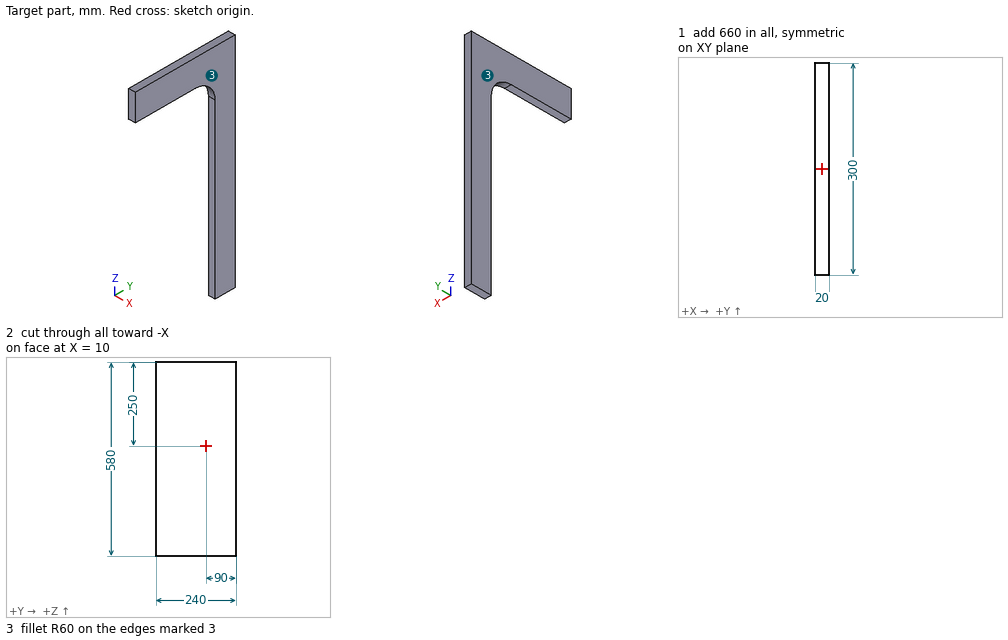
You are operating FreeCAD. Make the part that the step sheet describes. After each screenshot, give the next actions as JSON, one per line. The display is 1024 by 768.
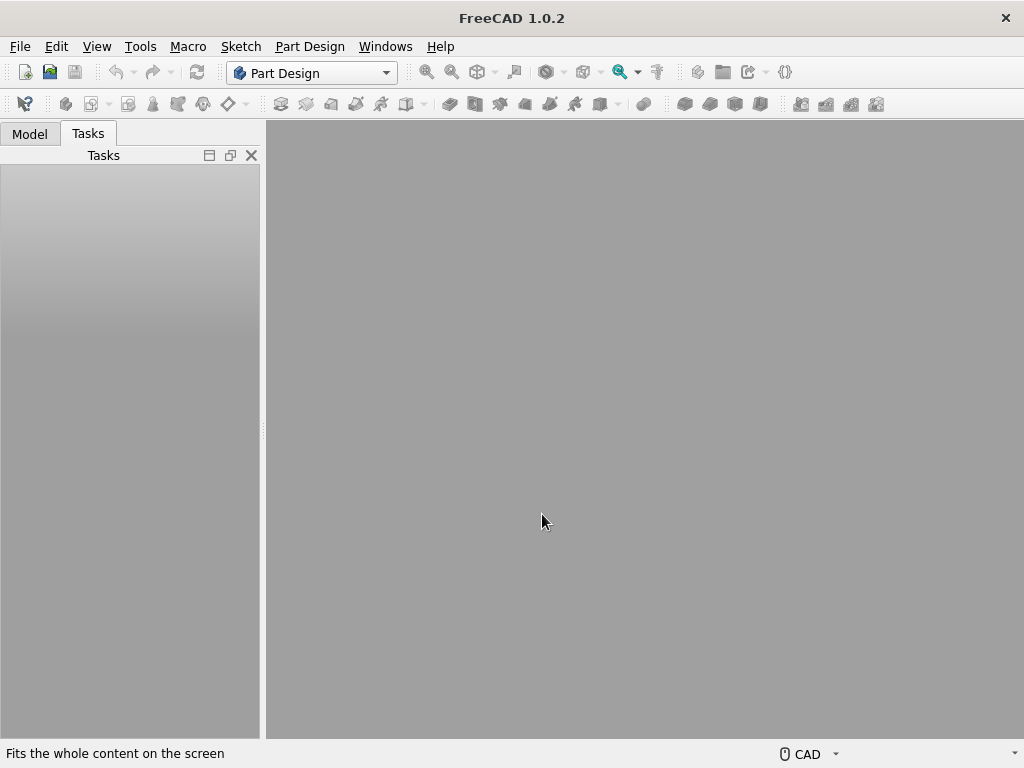
{"action": "key", "text": "ctrl+n"}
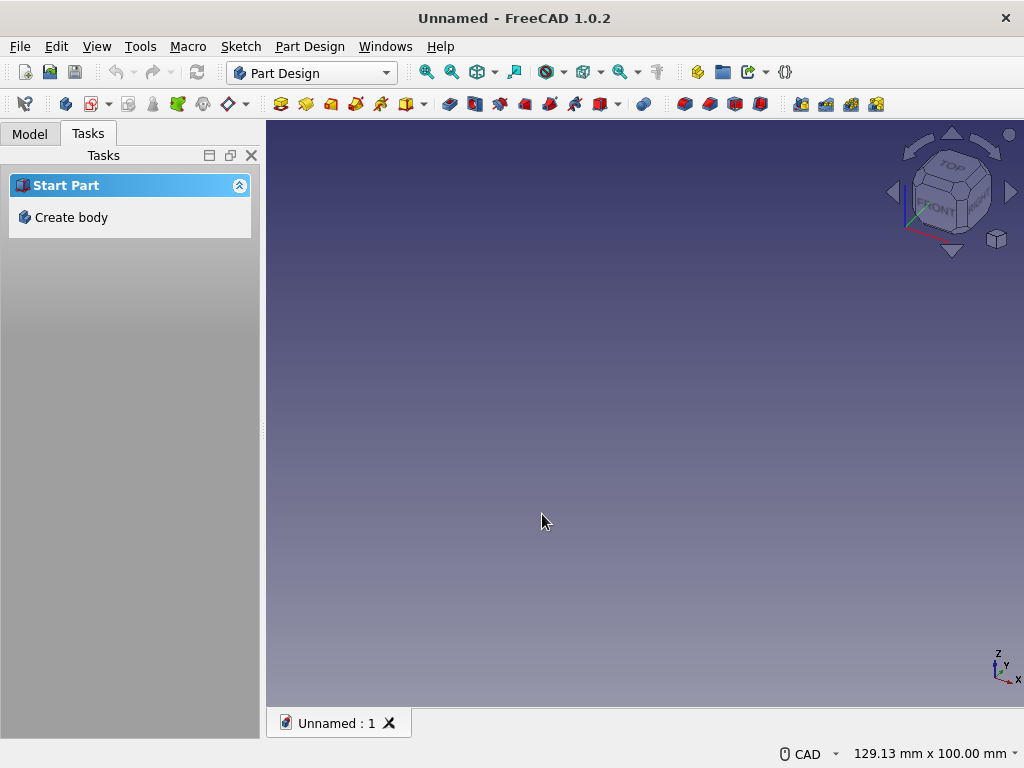
{"action": "left_click", "coordinate": [90, 104]}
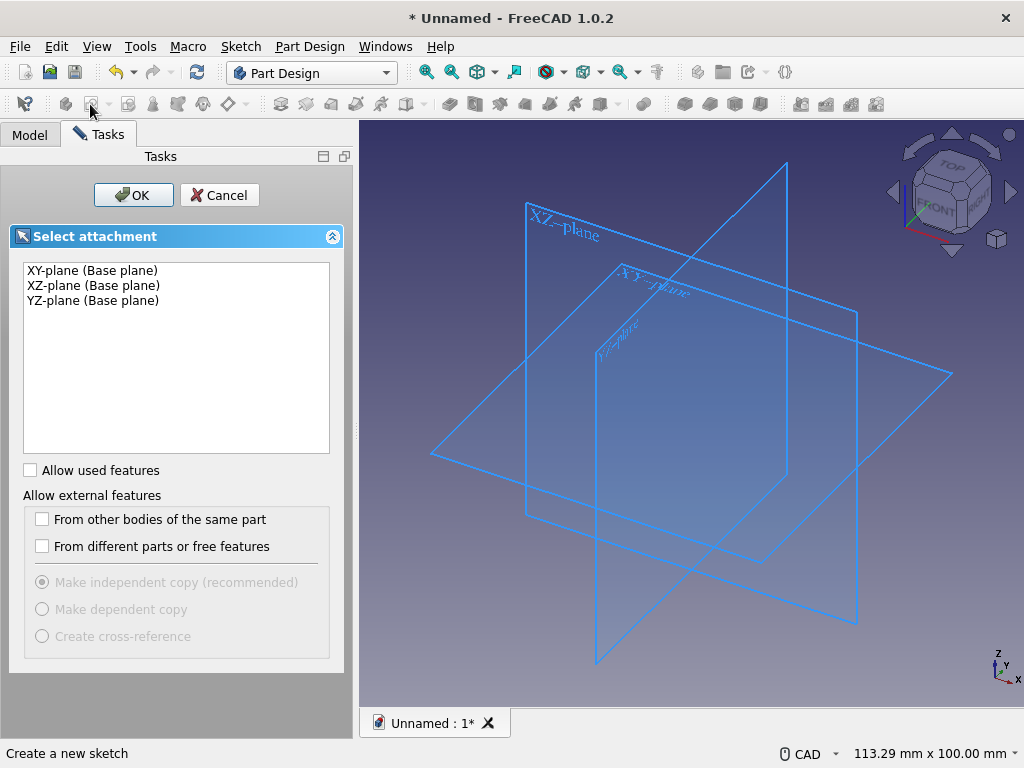
{"action": "left_click", "coordinate": [84, 270]}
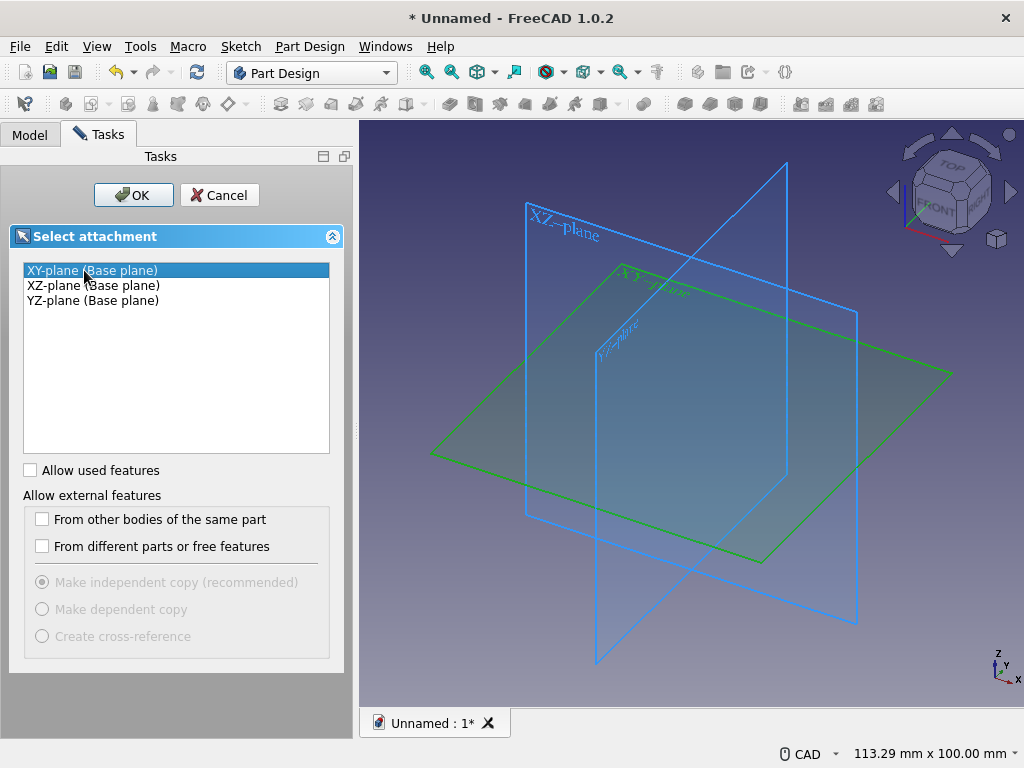
{"action": "left_click", "coordinate": [134, 195]}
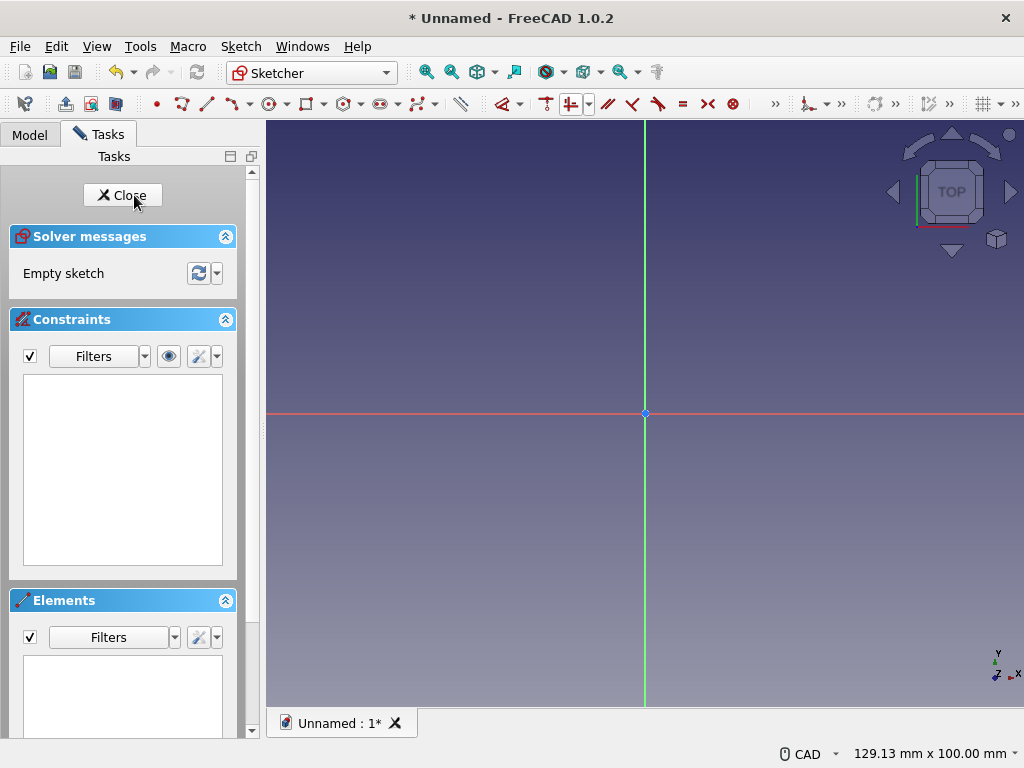
{"action": "scroll", "coordinate": [559, 414], "scroll_direction": "down", "scroll_amount": 8}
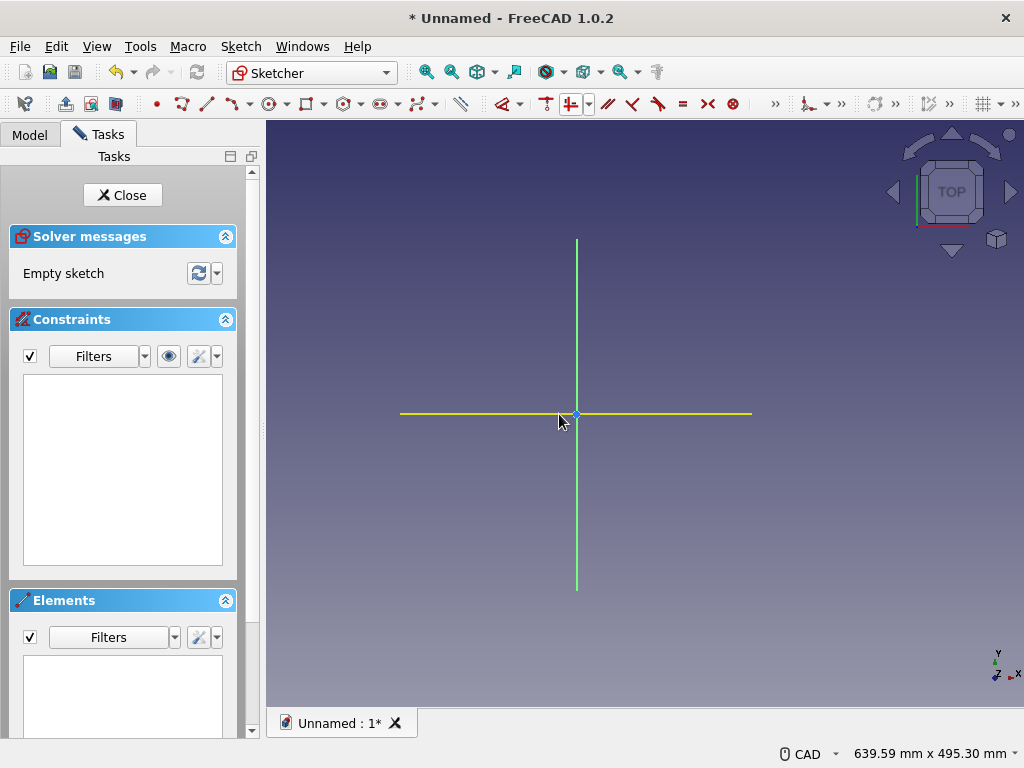
{"action": "left_click", "coordinate": [324, 104]}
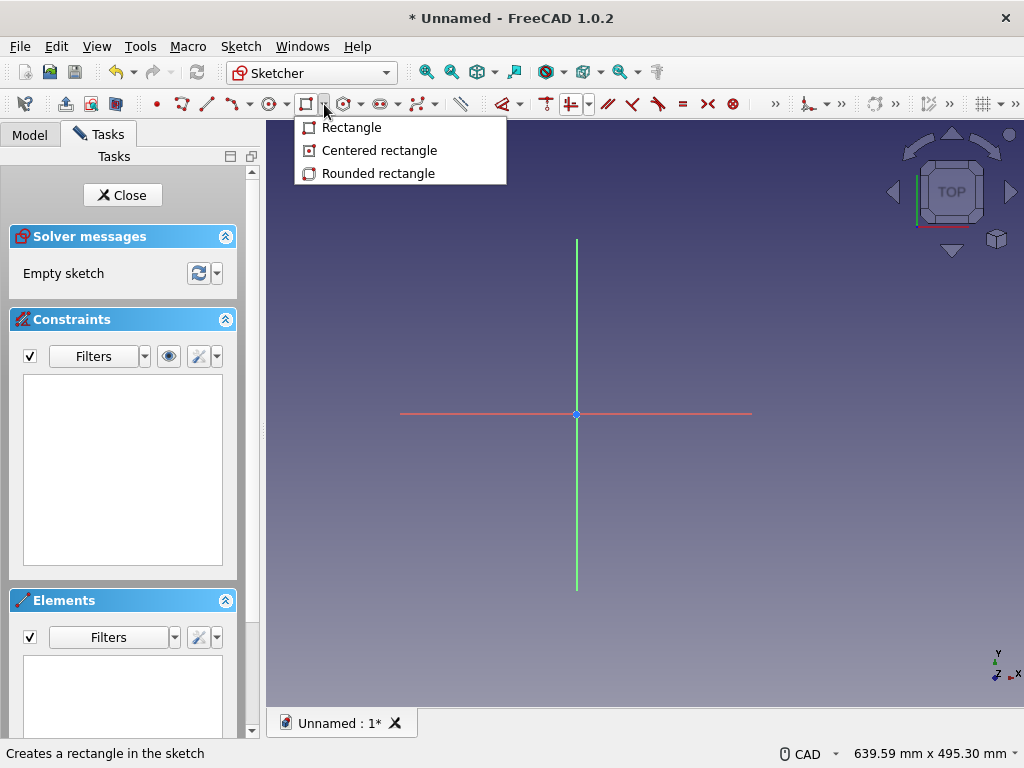
{"action": "left_click", "coordinate": [400, 150]}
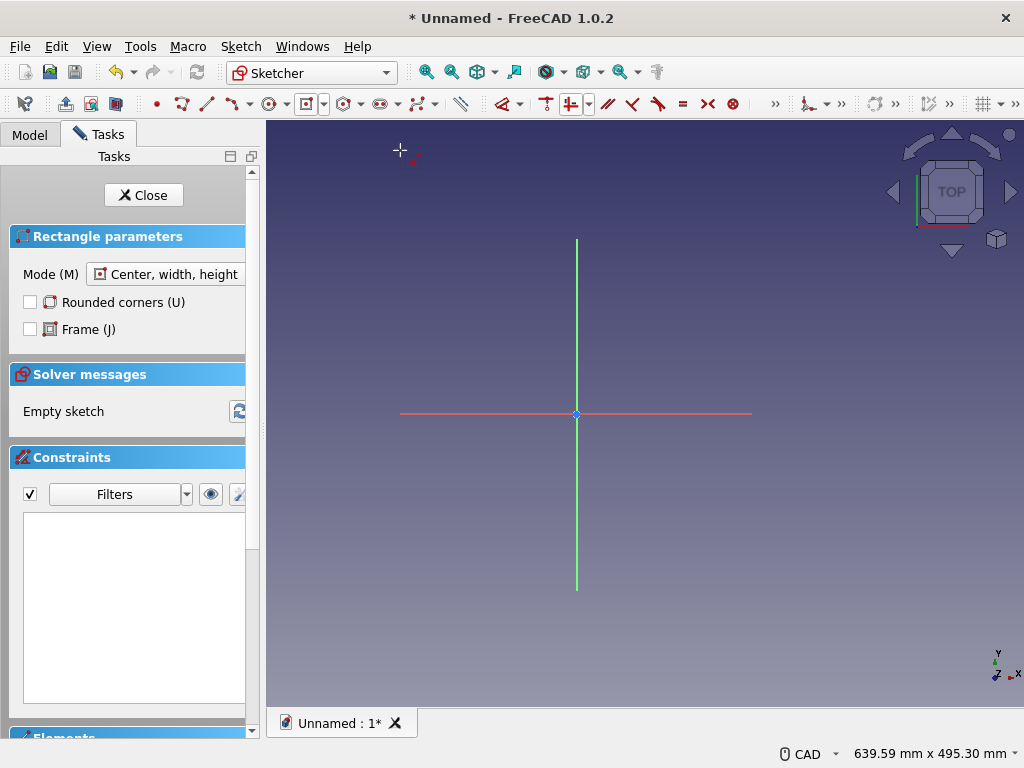
{"action": "scroll", "coordinate": [577, 414], "scroll_direction": "up", "scroll_amount": 2}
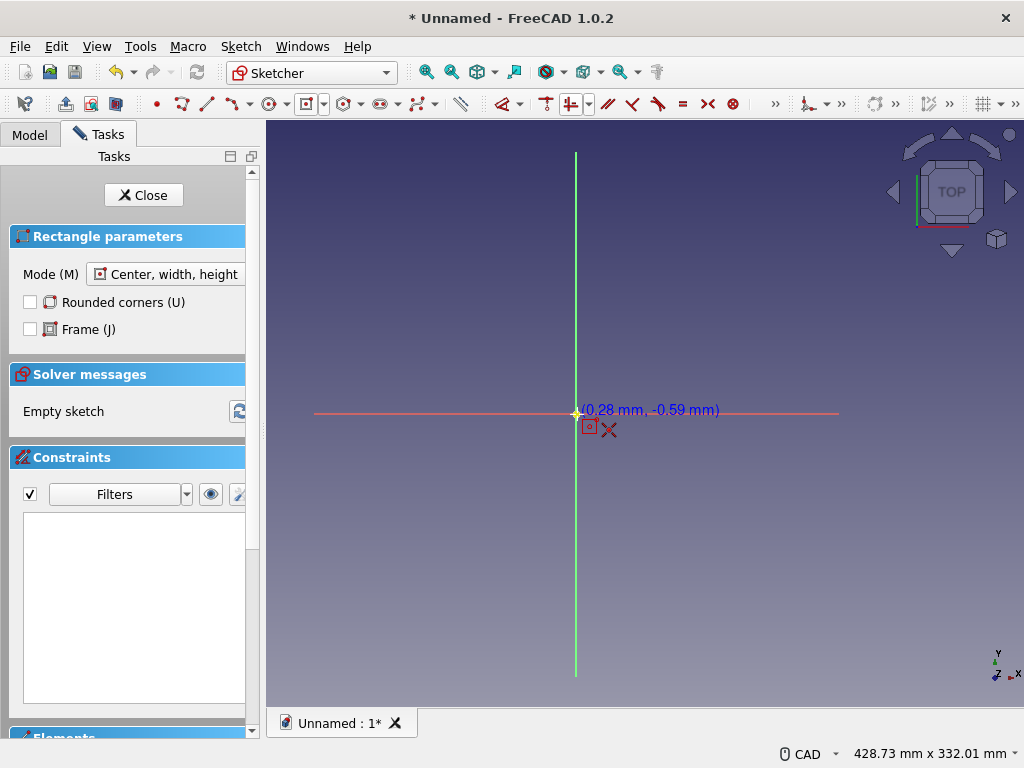
{"action": "left_click", "coordinate": [576, 414]}
{"action": "left_click", "coordinate": [594, 149]}
{"action": "key", "text": "Escape"}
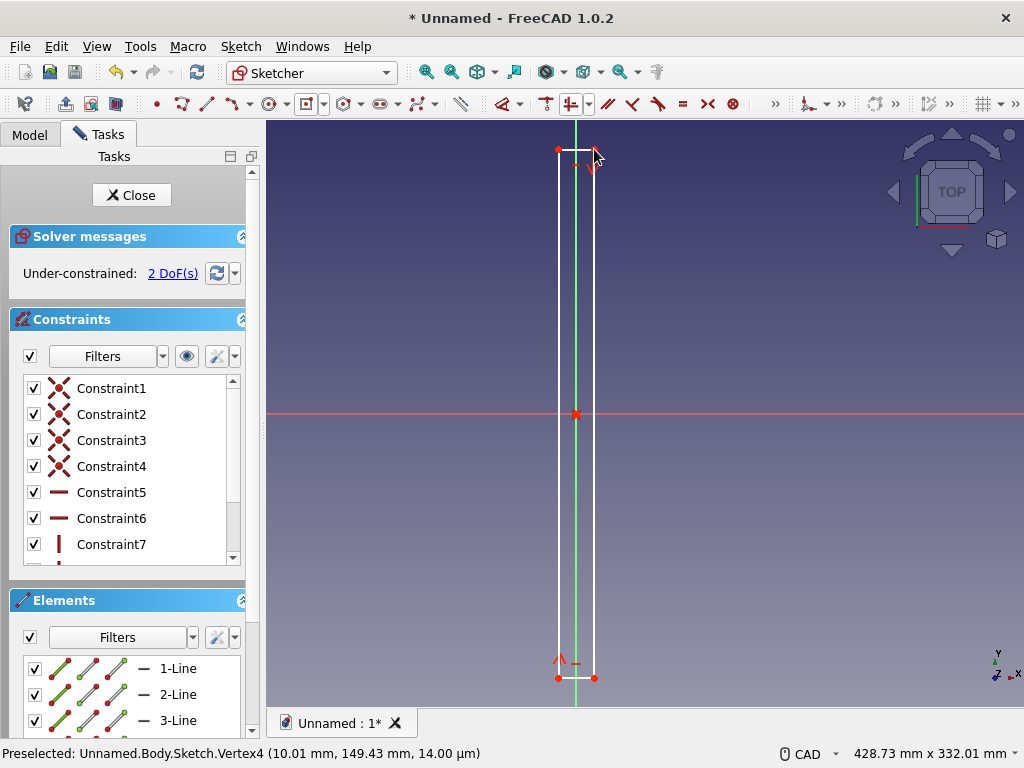
{"action": "left_click", "coordinate": [502, 104]}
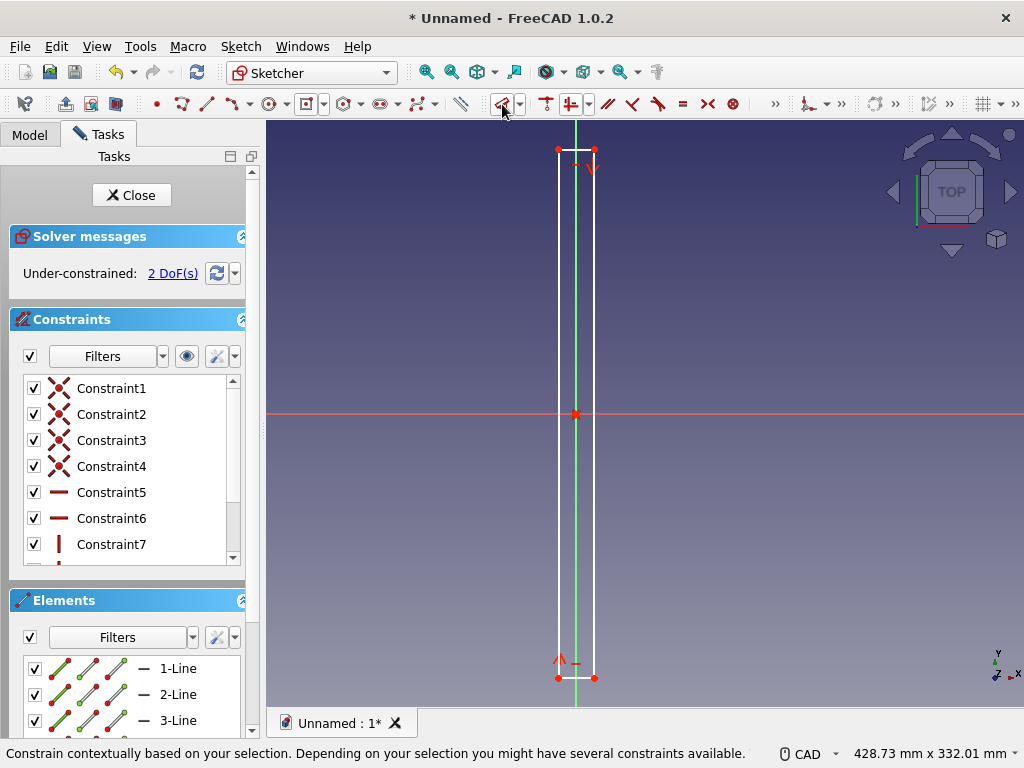
{"action": "left_click", "coordinate": [573, 678]}
{"action": "left_click", "coordinate": [568, 644]}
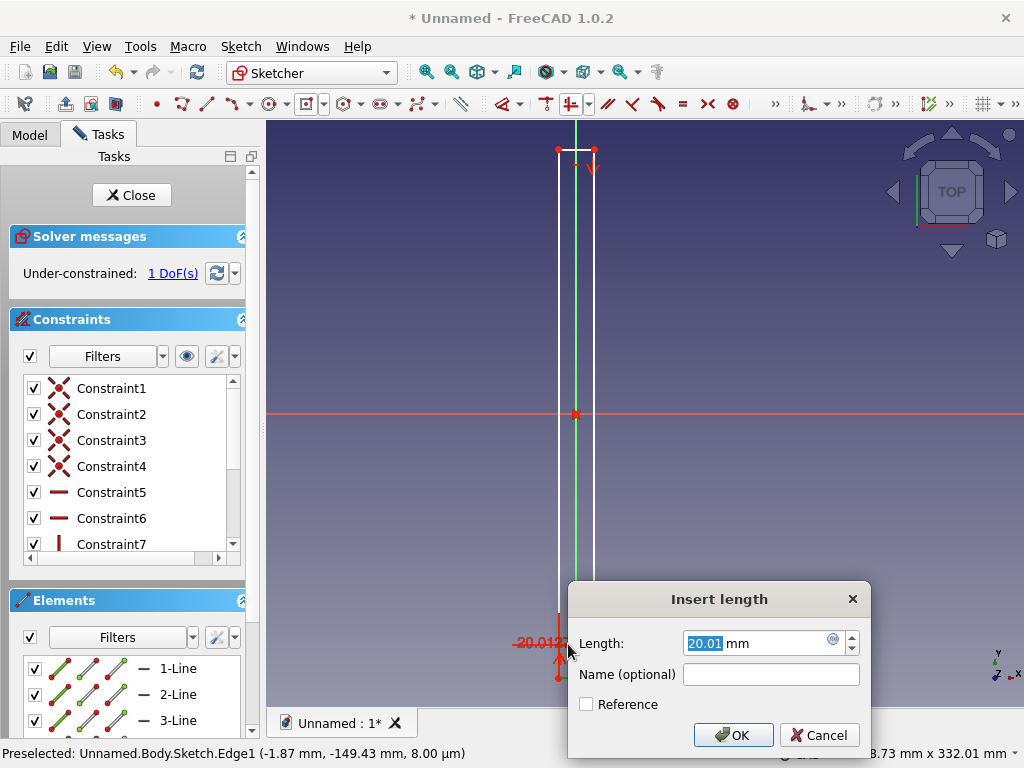
{"action": "type", "text": "20"}
{"action": "key", "text": "Return"}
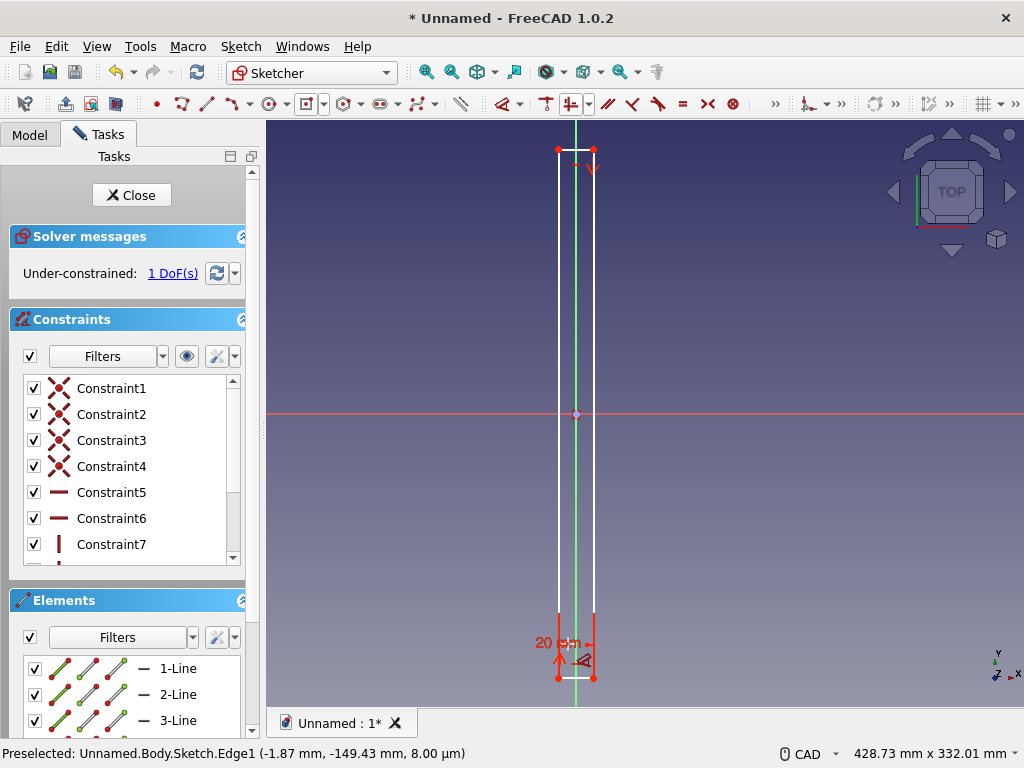
{"action": "left_click", "coordinate": [594, 520]}
{"action": "left_click", "coordinate": [628, 293]}